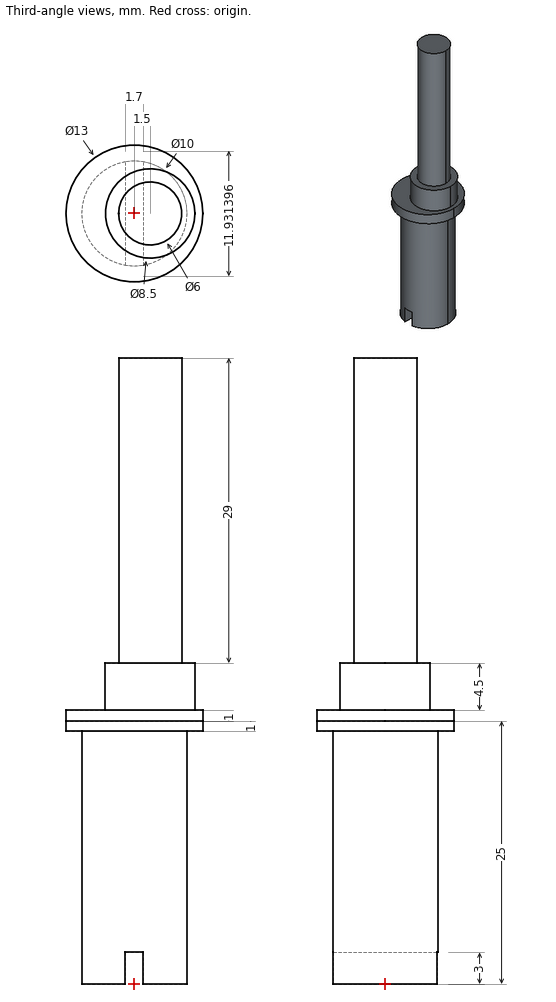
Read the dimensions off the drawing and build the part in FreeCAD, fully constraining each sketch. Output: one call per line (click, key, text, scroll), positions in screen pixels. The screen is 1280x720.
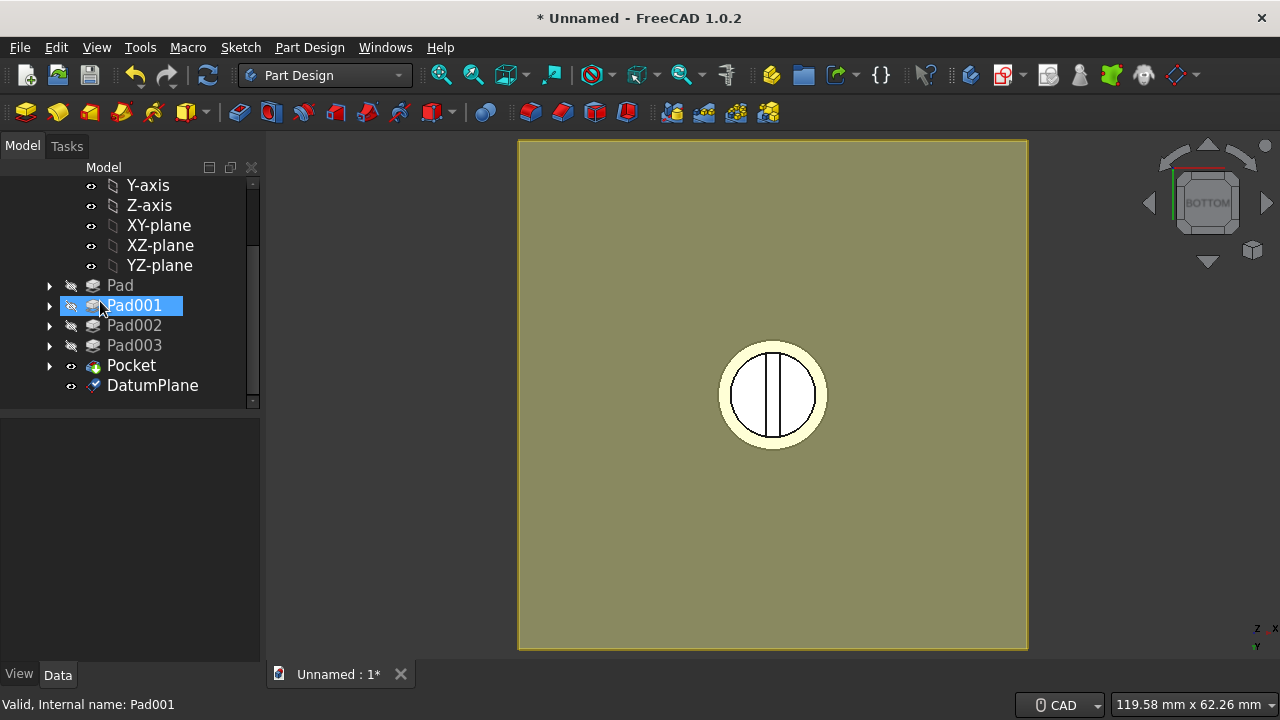
click(116, 386)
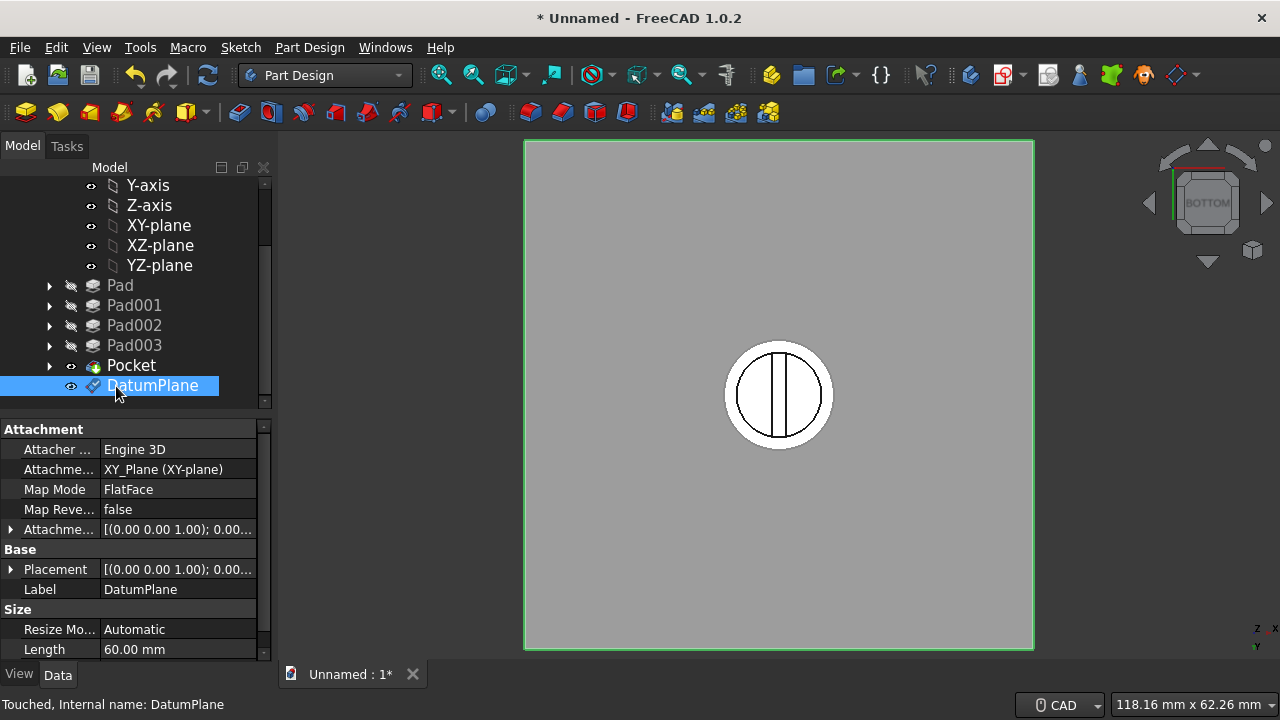
click(1004, 76)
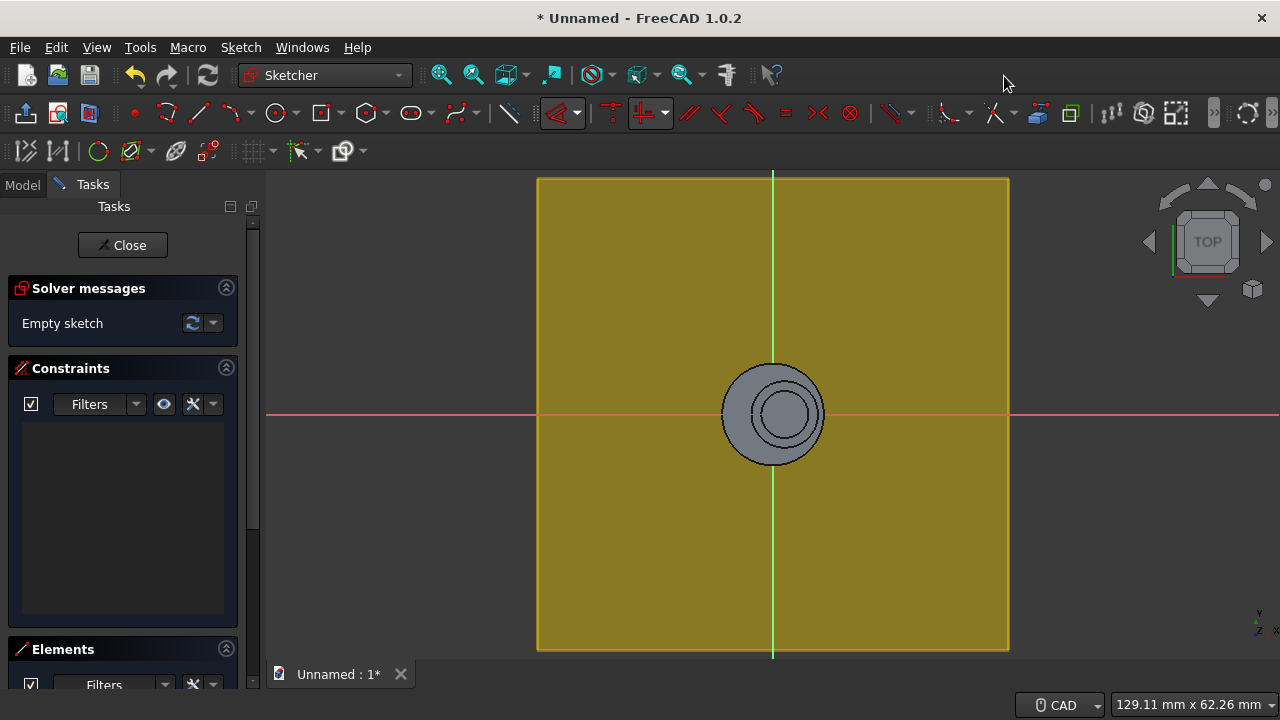
click(90, 114)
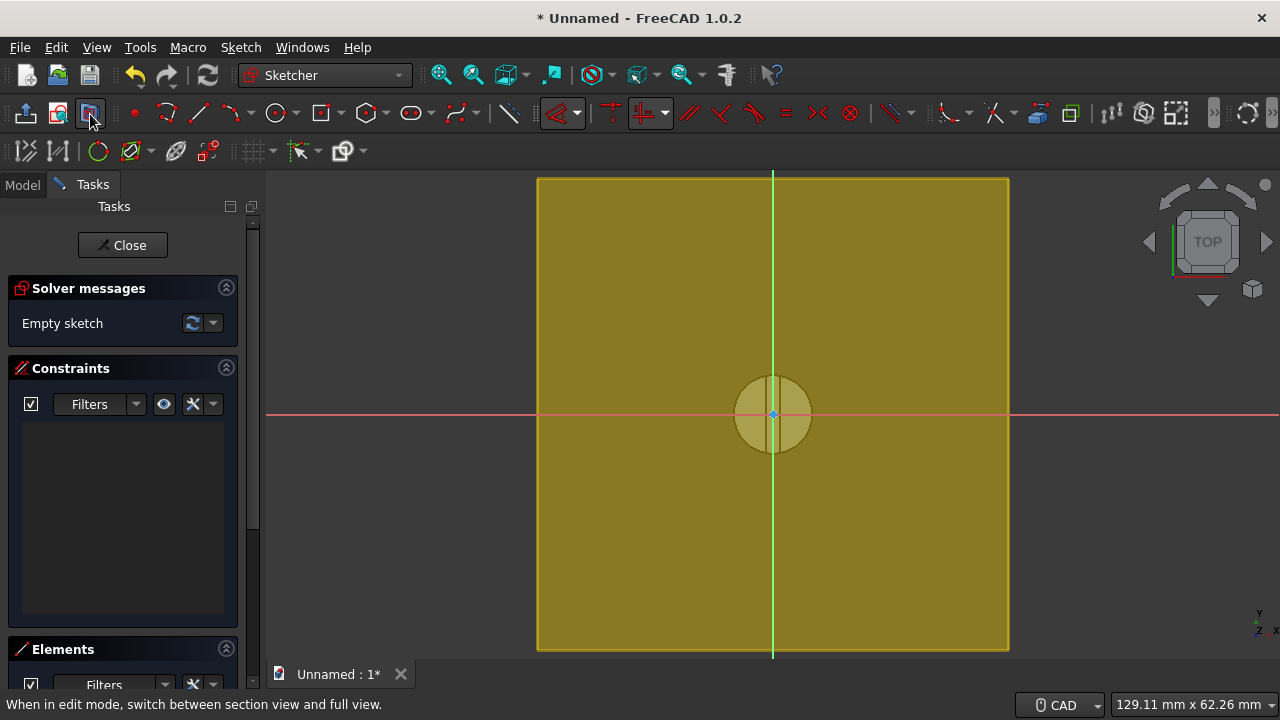
scroll(813, 415, up, 5)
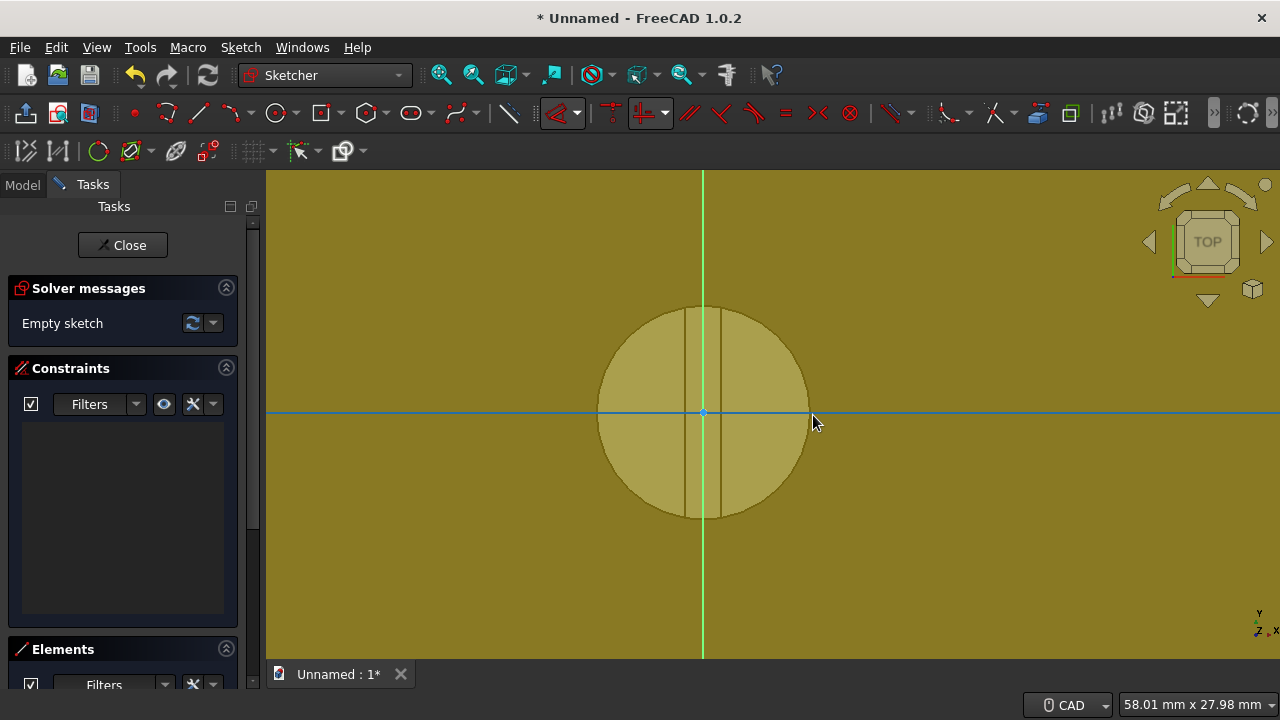
click(276, 114)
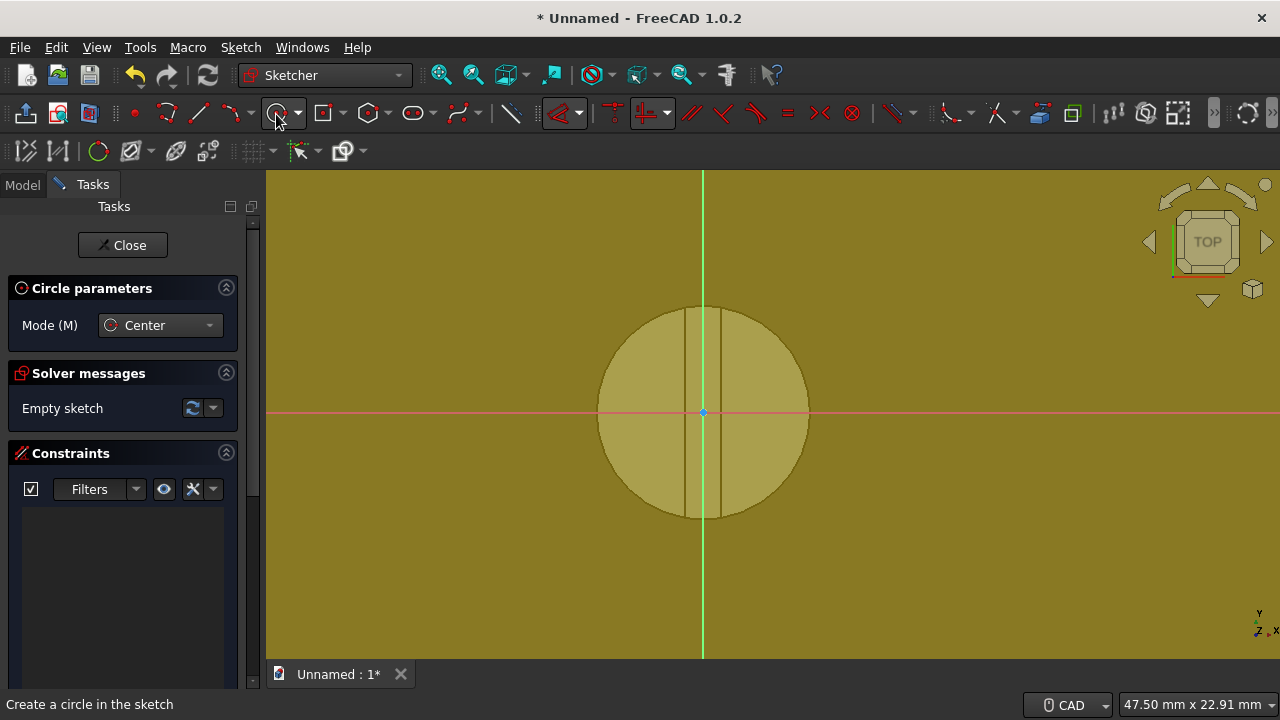
click(703, 413)
move(801, 315)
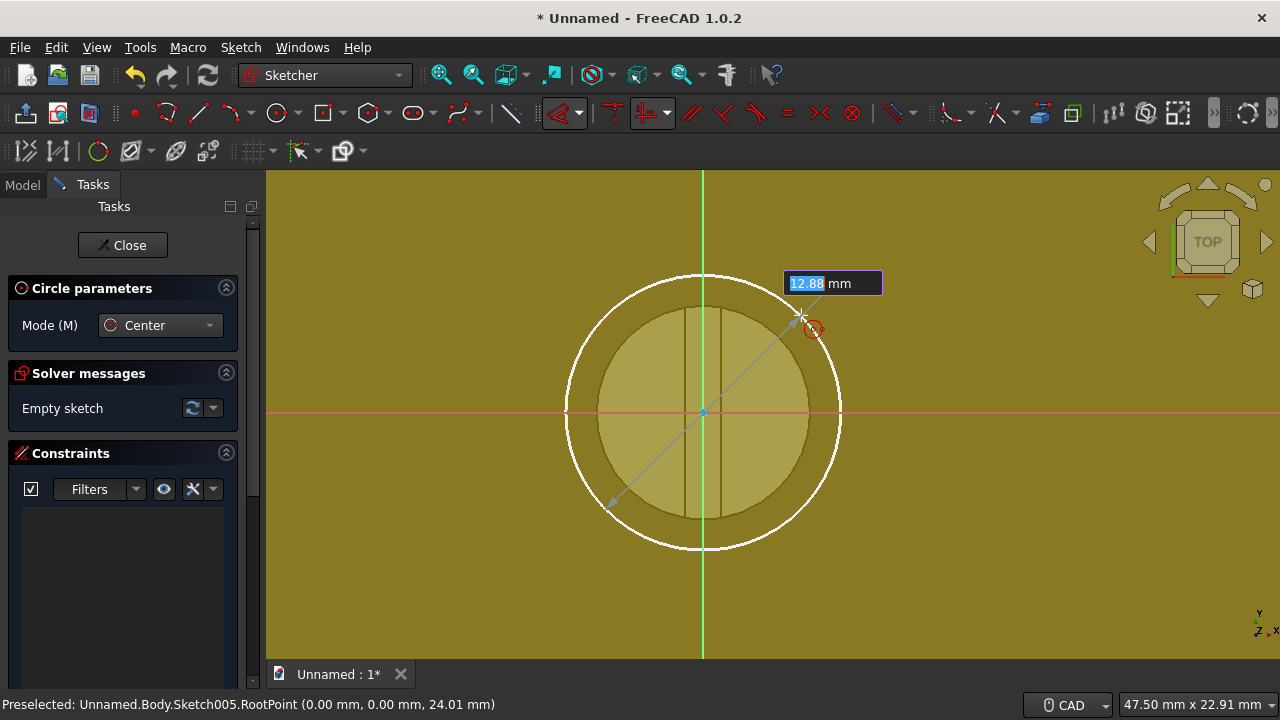
text(13)
key(Return)
key(Escape)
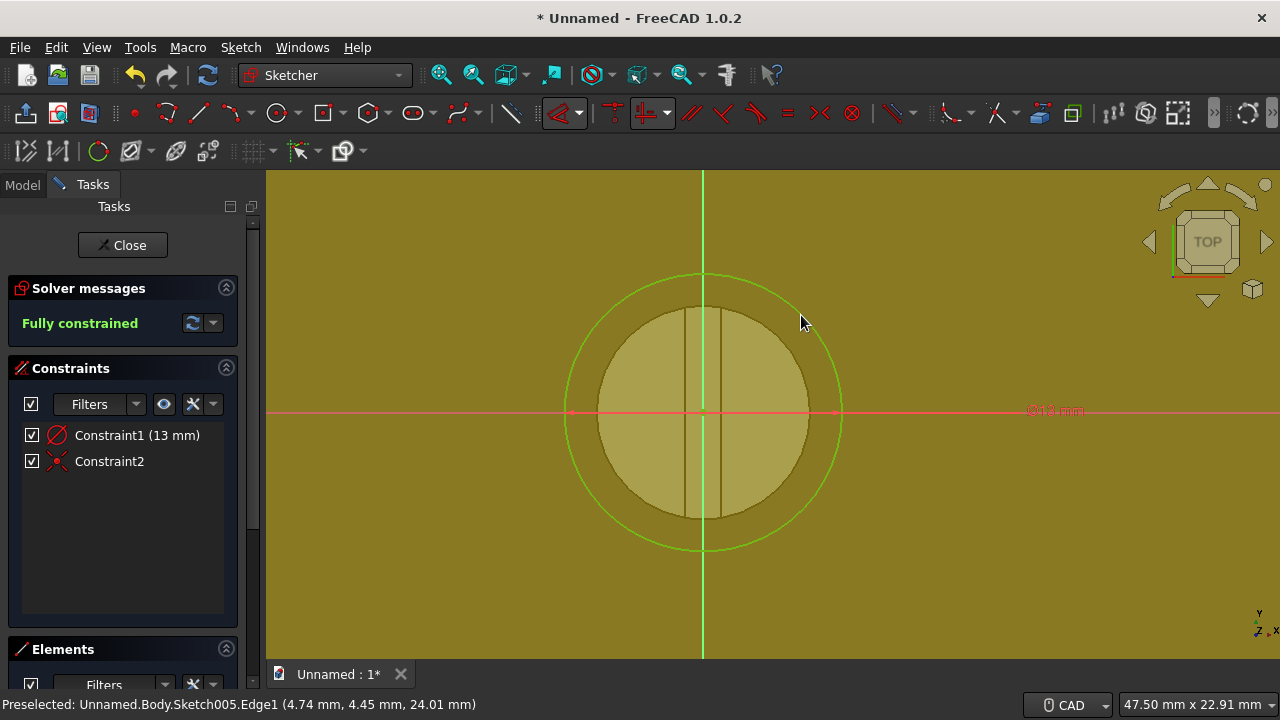
click(123, 245)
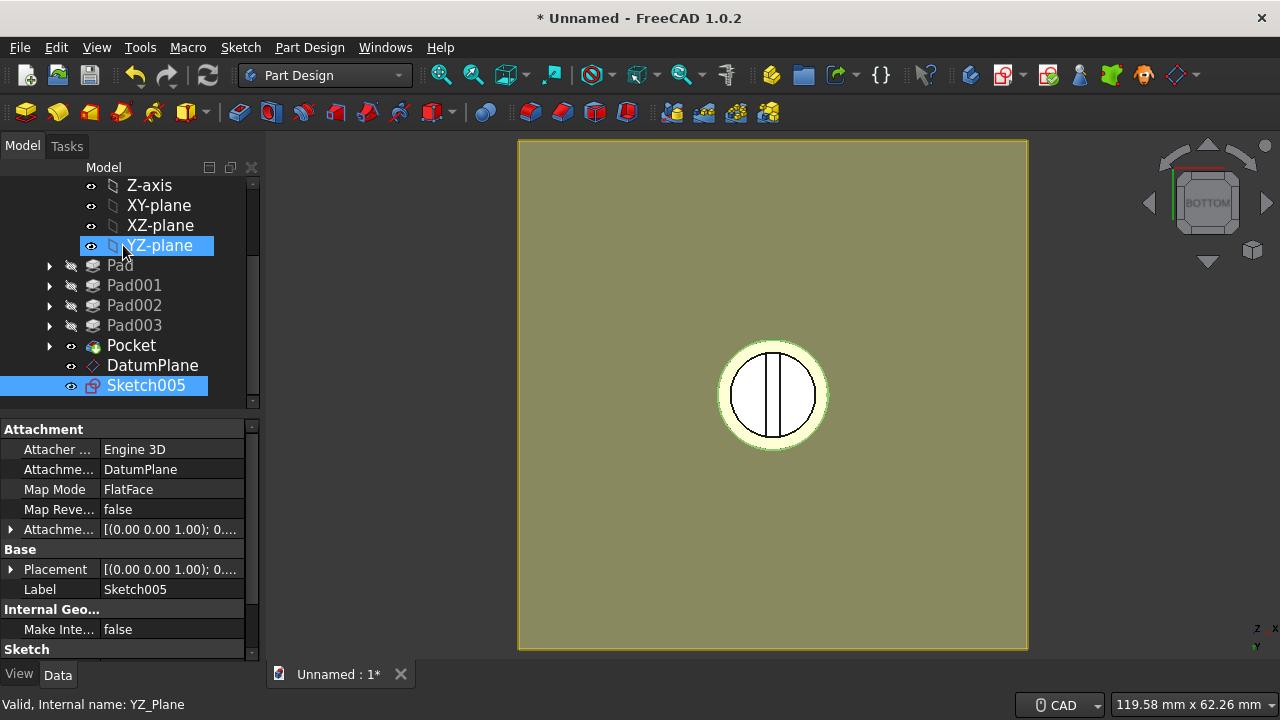
click(26, 112)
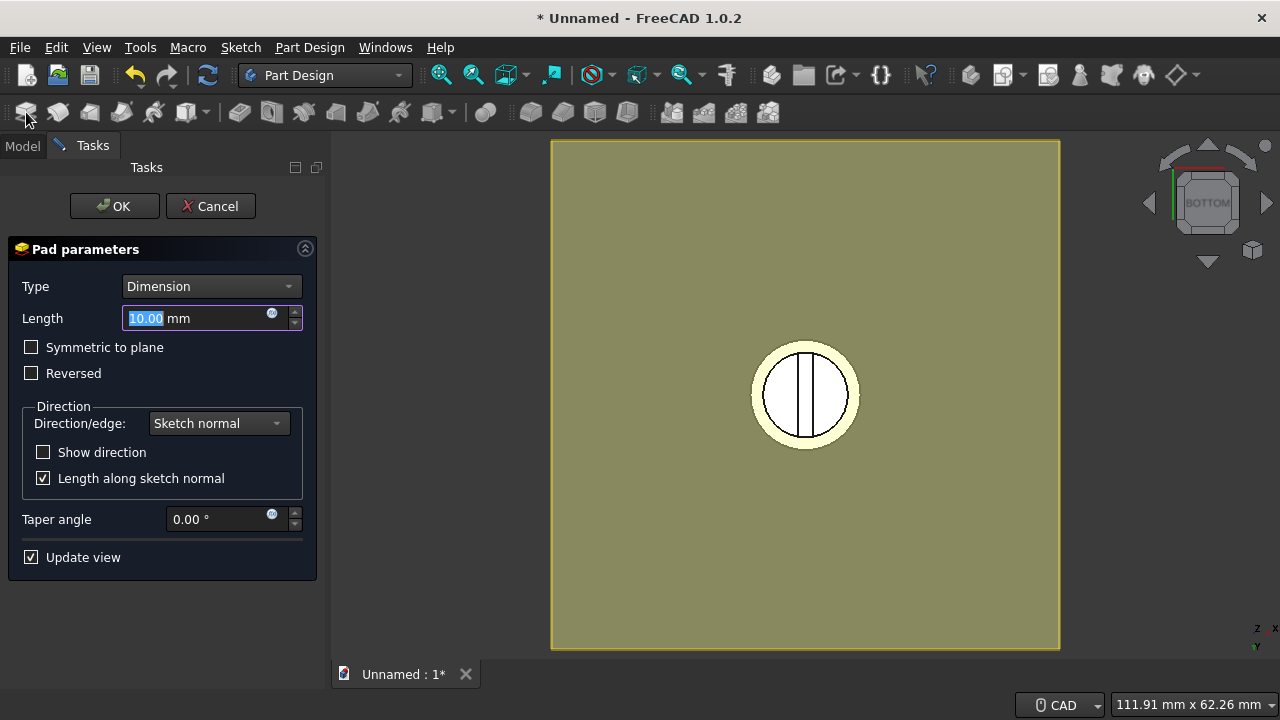
text(1)
key(Tab)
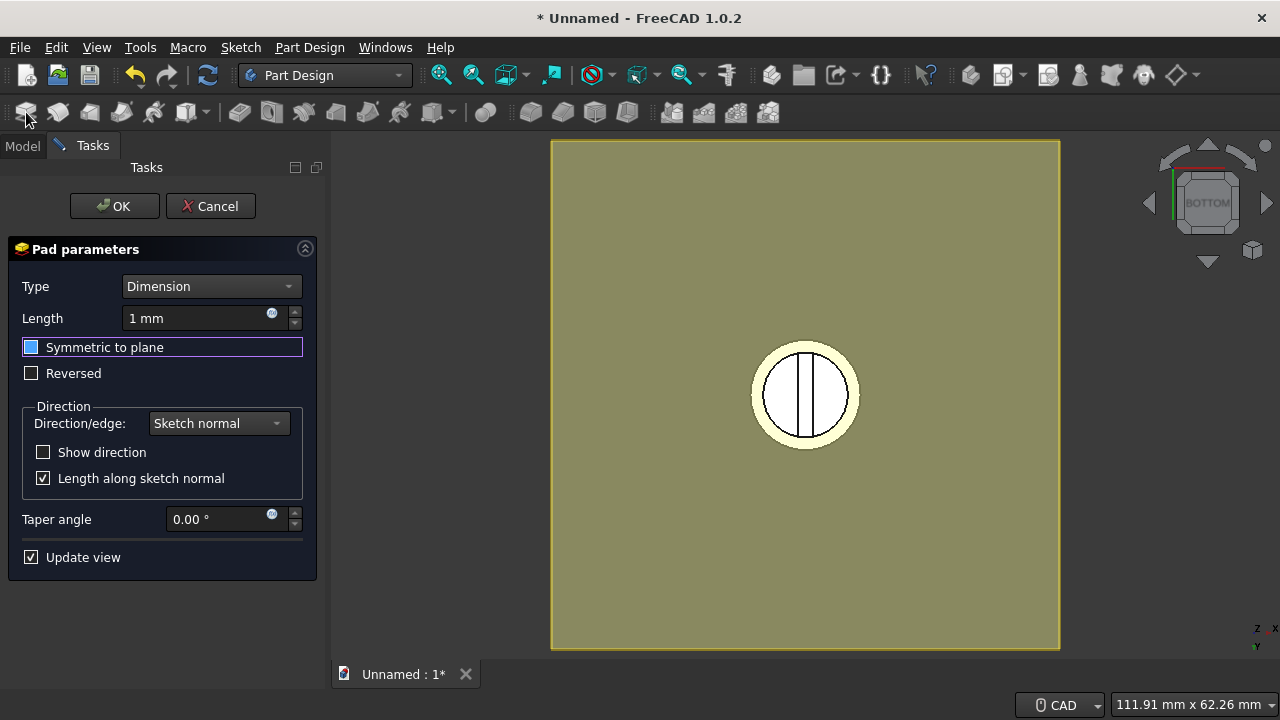
click(115, 206)